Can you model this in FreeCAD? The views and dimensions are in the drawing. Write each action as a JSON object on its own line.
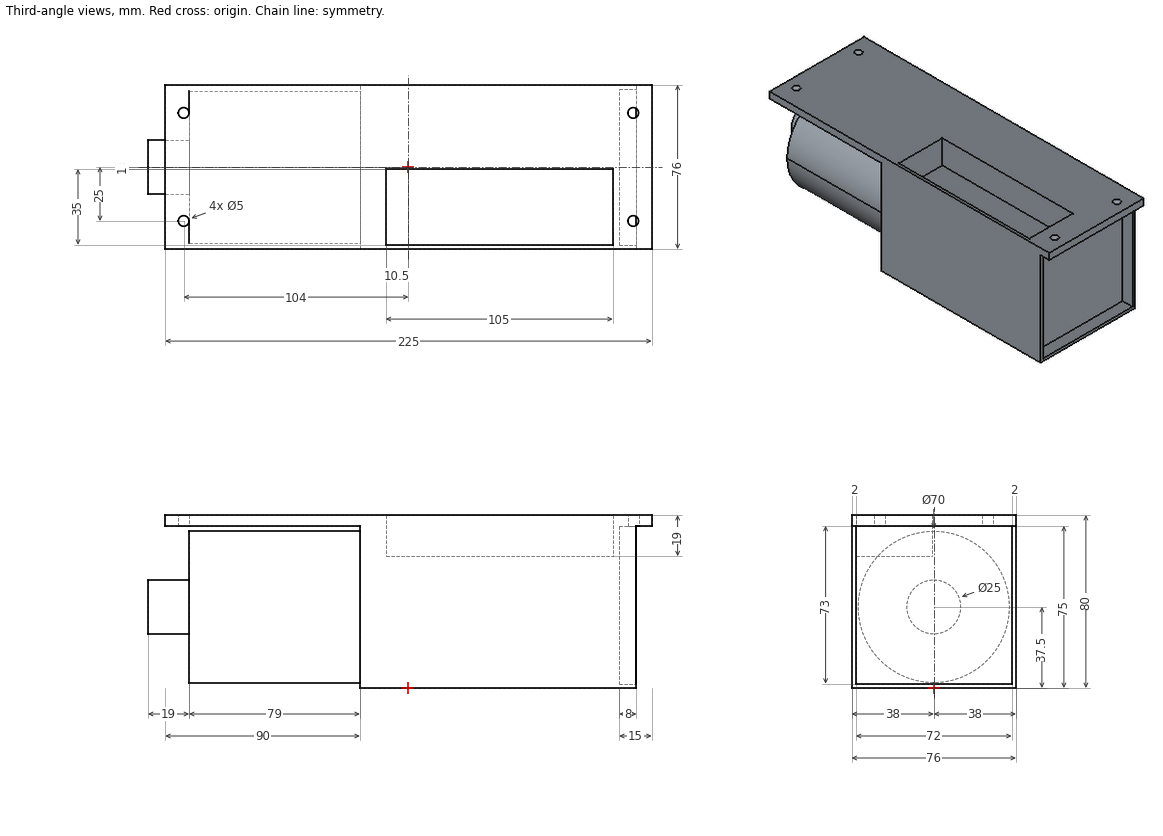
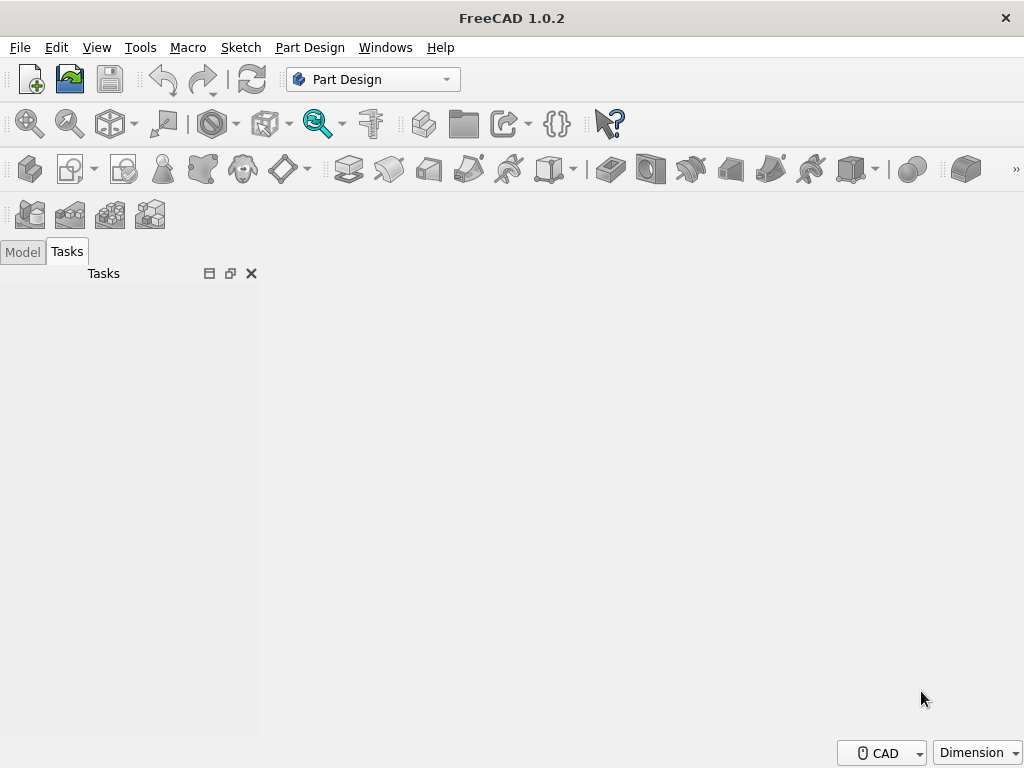
{"action": "key", "text": "ctrl+n"}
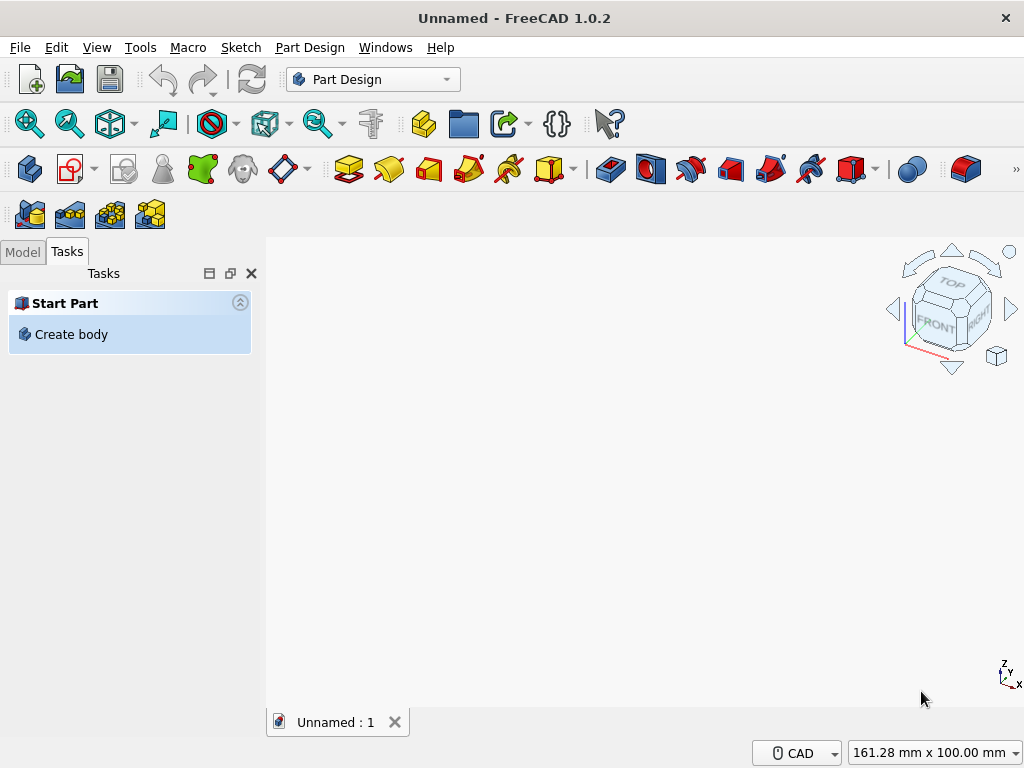
{"action": "left_click", "coordinate": [70, 170]}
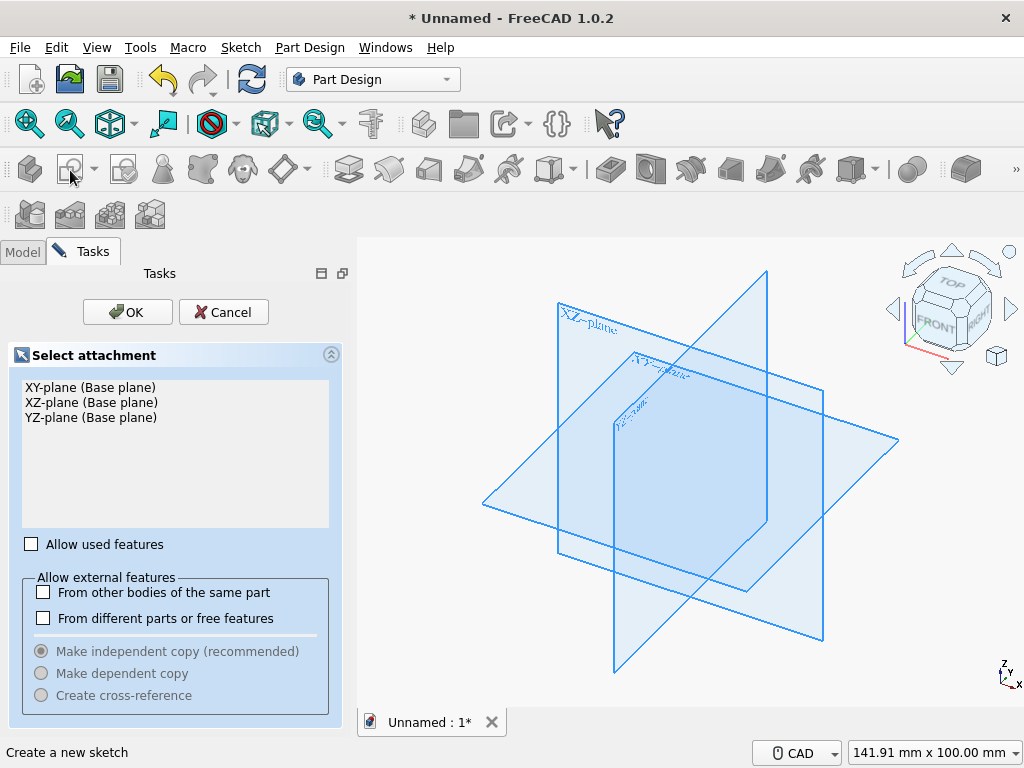
{"action": "left_click", "coordinate": [82, 388]}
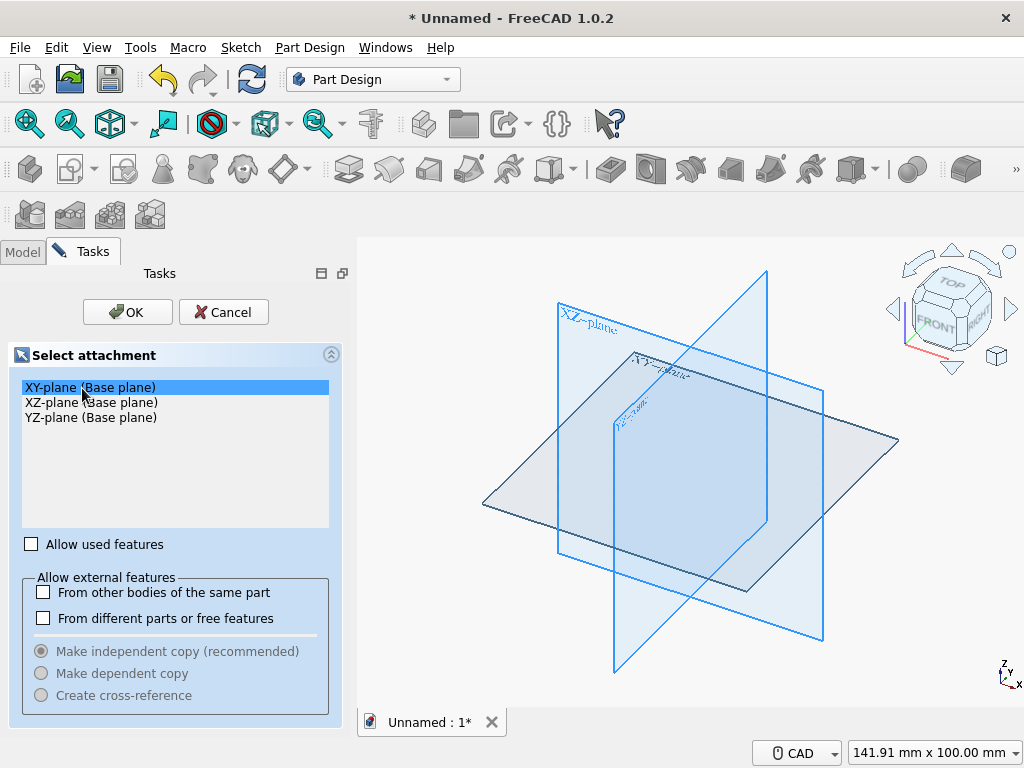
{"action": "left_click", "coordinate": [128, 312]}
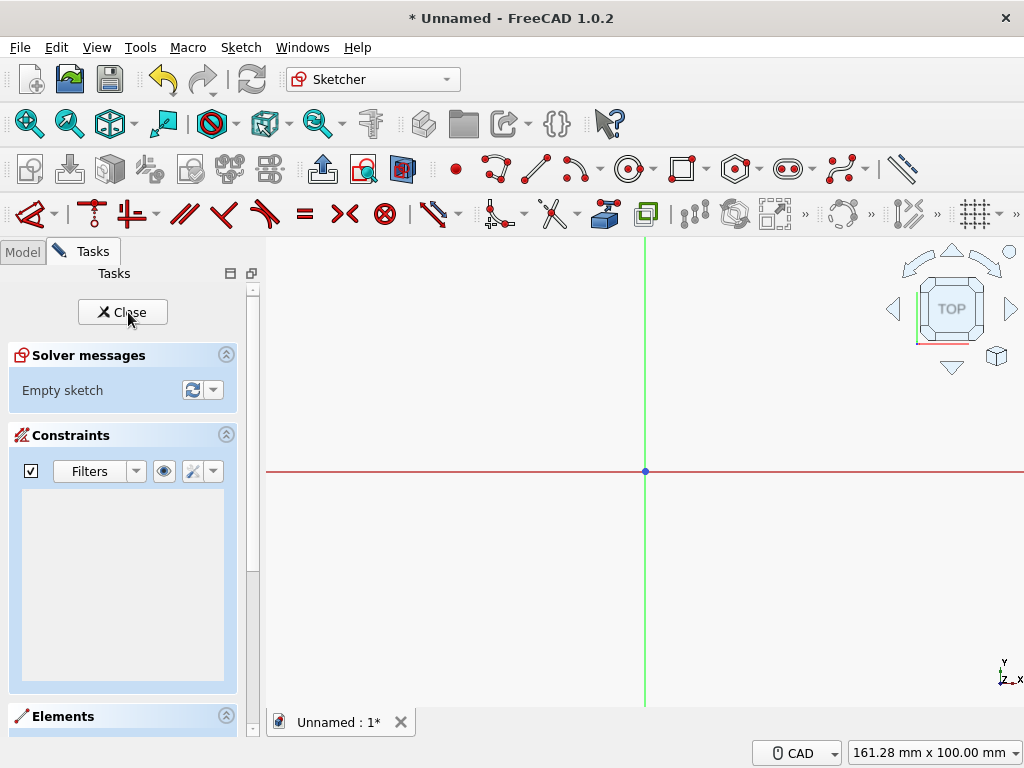
{"action": "scroll", "coordinate": [537, 472], "scroll_direction": "down", "scroll_amount": 5}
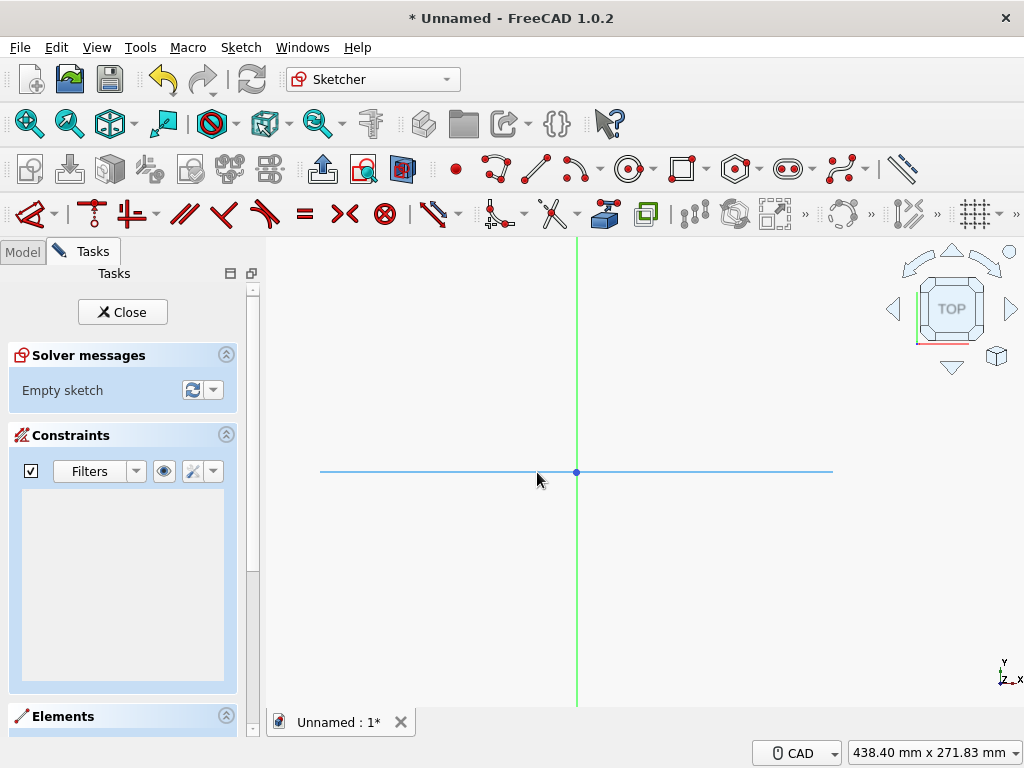
{"action": "key", "text": "g v"}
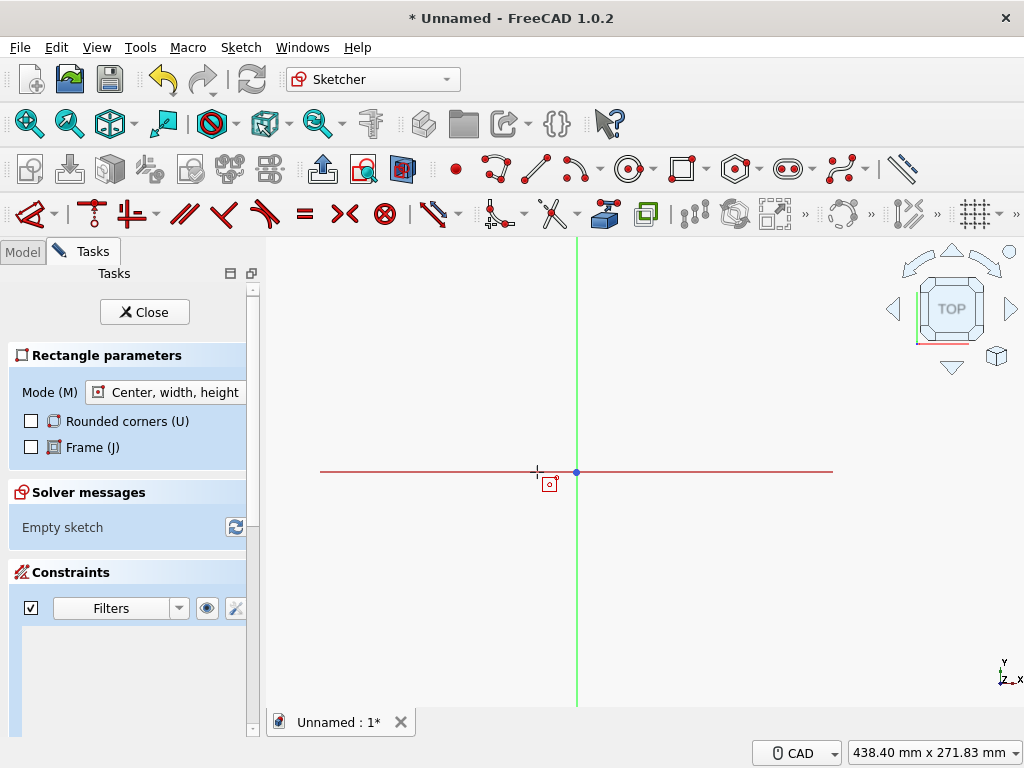
{"action": "left_click", "coordinate": [577, 472]}
{"action": "left_click", "coordinate": [771, 407]}
{"action": "key", "text": "Escape"}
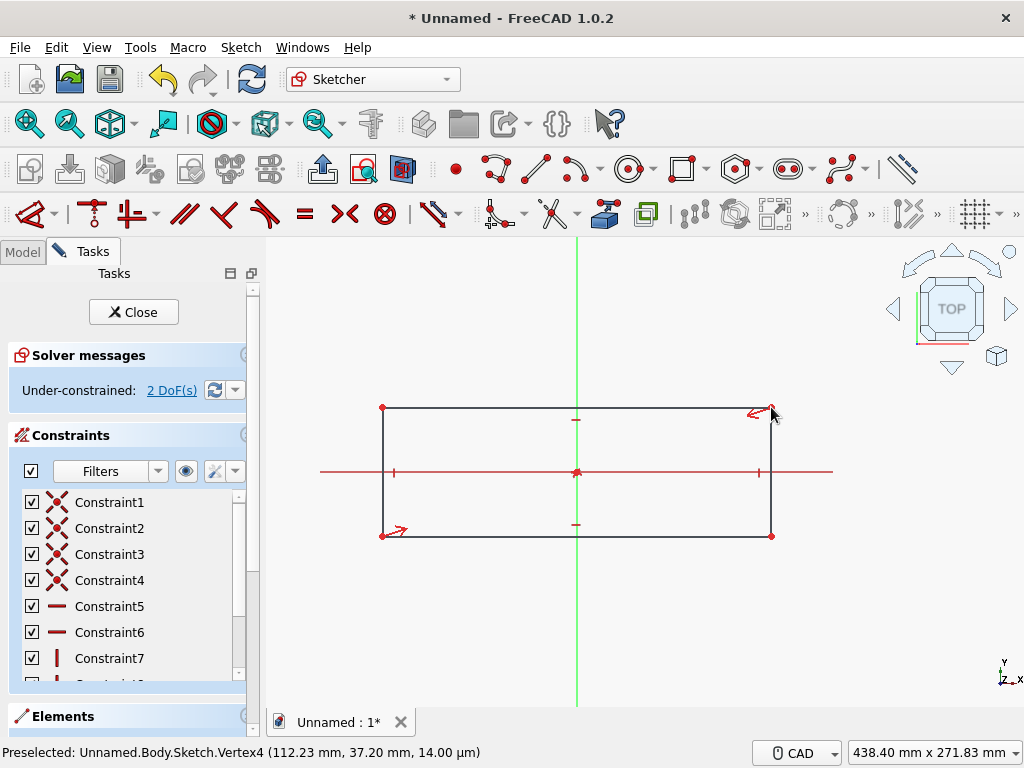
{"action": "key", "text": "d"}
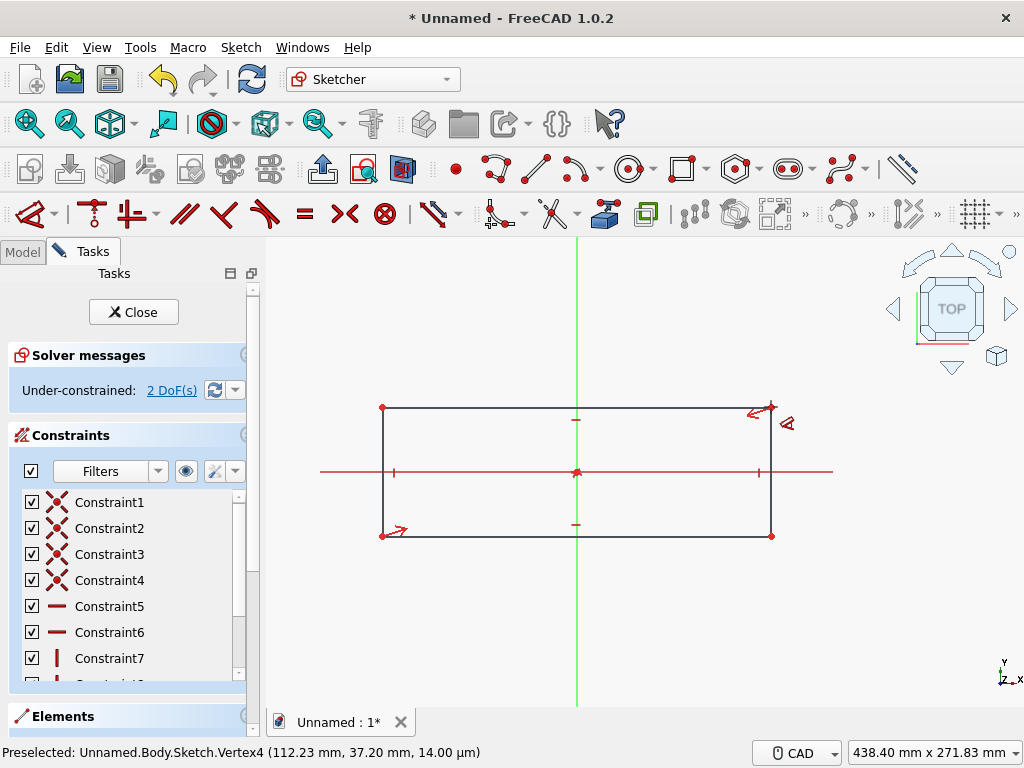
{"action": "left_click", "coordinate": [771, 498]}
{"action": "left_click", "coordinate": [805, 443]}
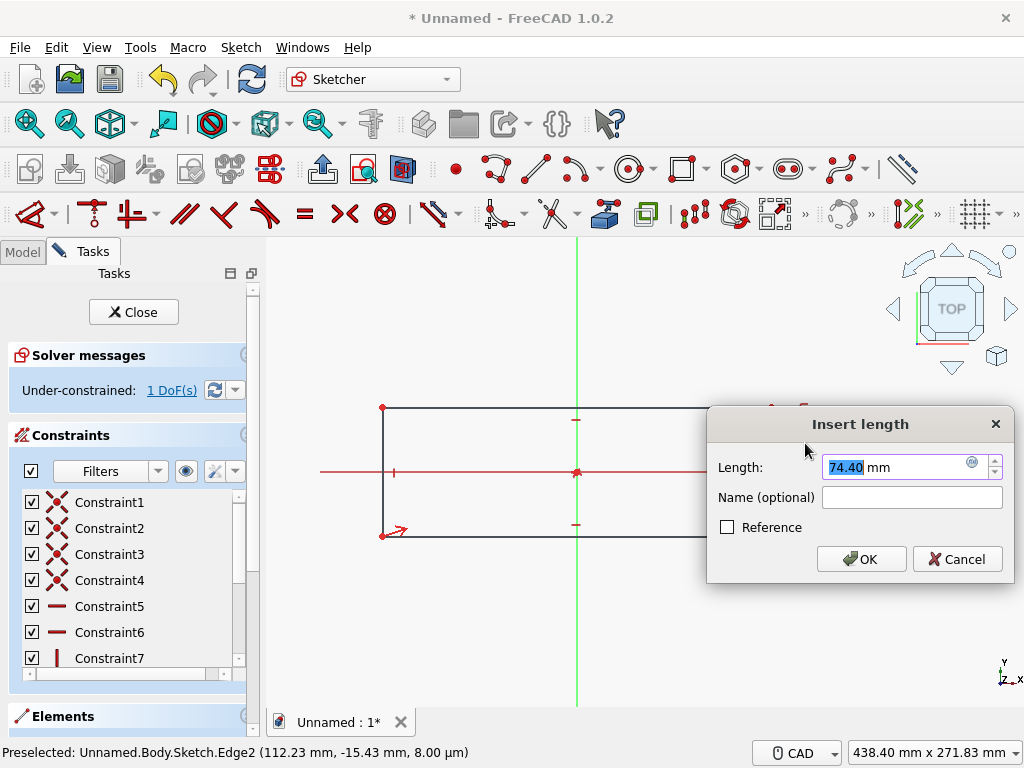
{"action": "type", "text": "76"}
{"action": "key", "text": "Return"}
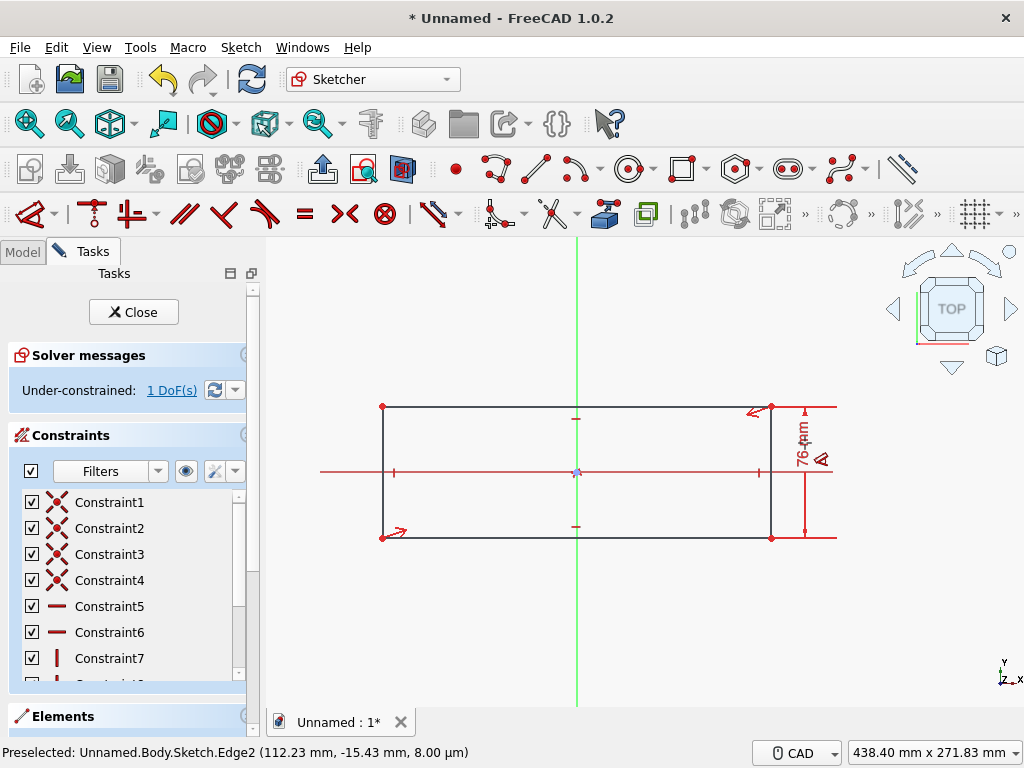
{"action": "left_click", "coordinate": [499, 538]}
{"action": "left_click", "coordinate": [488, 572]}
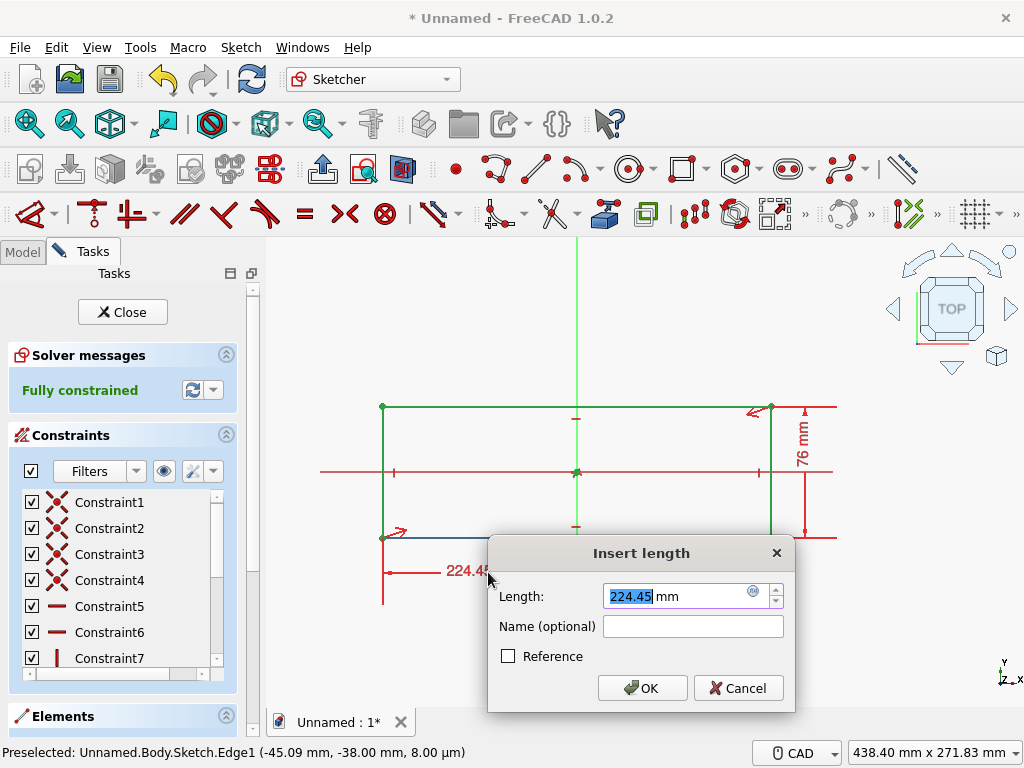
{"action": "type", "text": "225"}
{"action": "key", "text": "Return"}
{"action": "key", "text": "Escape"}